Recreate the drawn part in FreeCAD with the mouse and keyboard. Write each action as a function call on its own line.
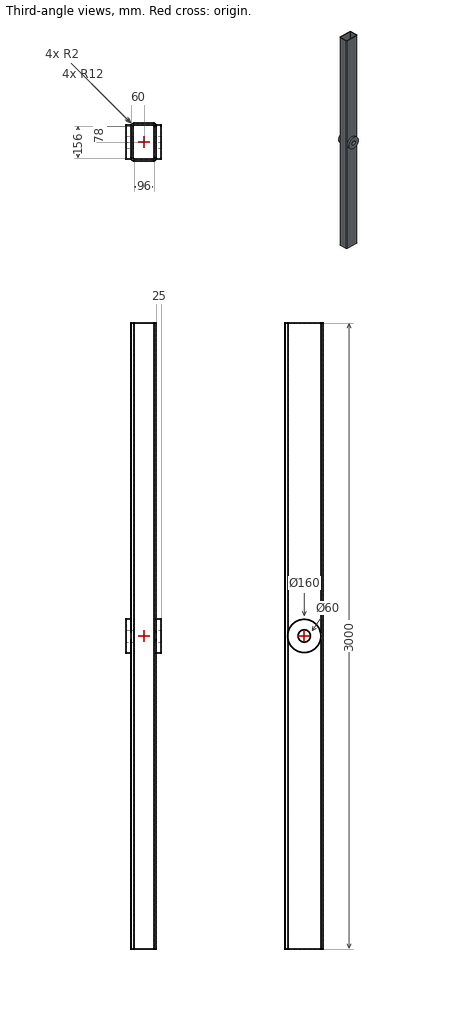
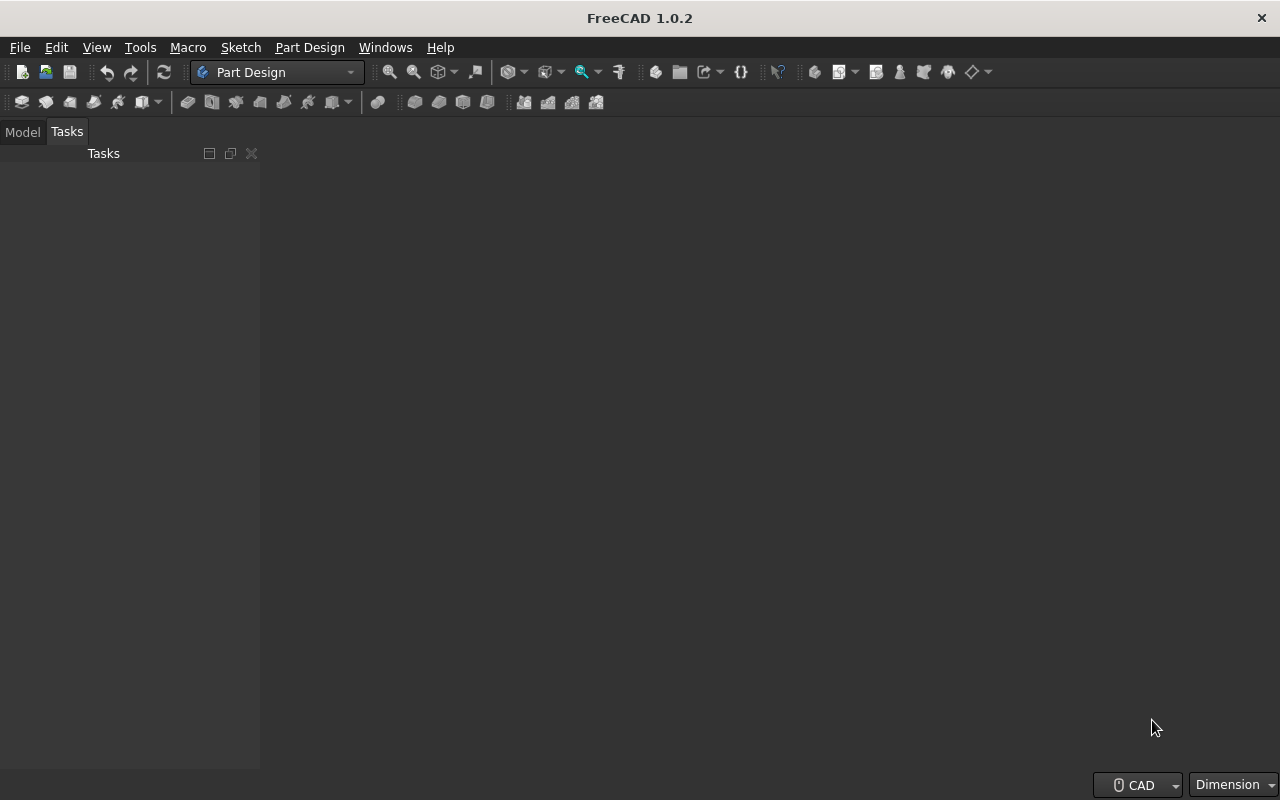
click(22, 72)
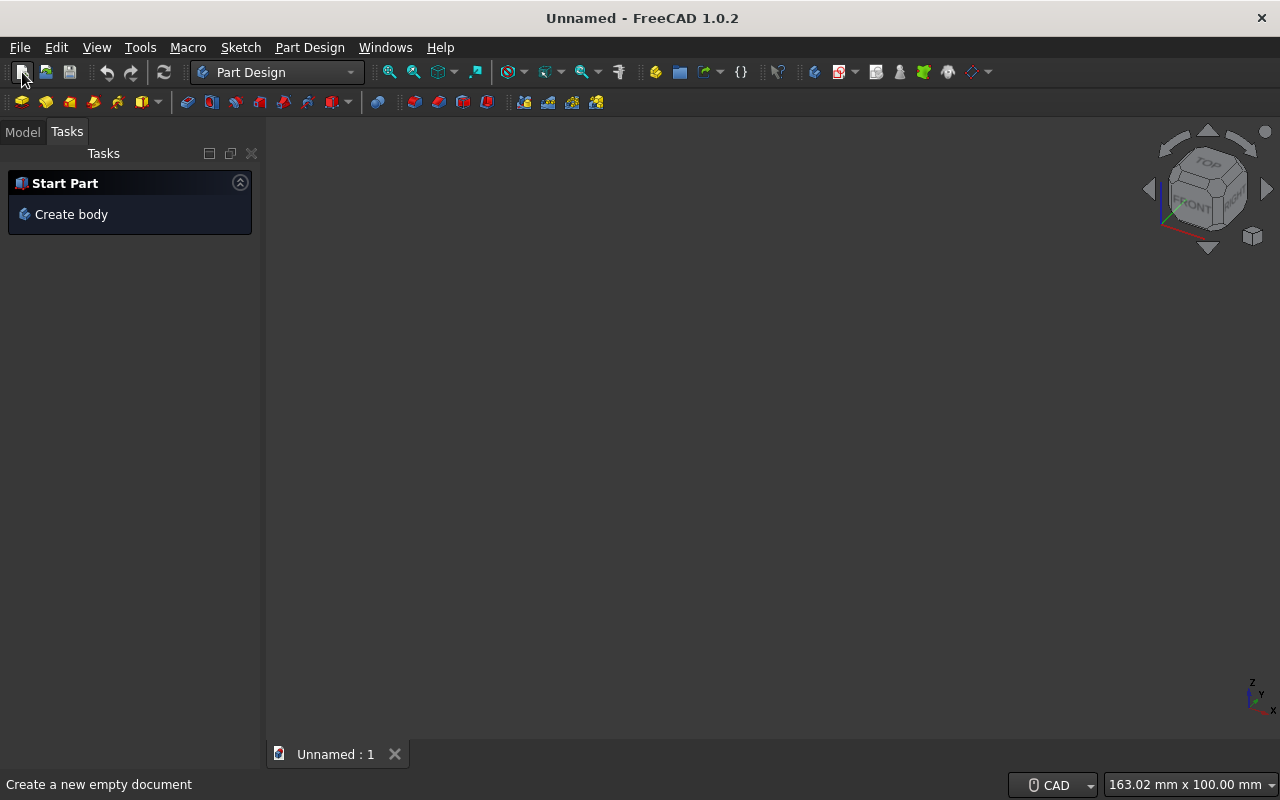
click(840, 72)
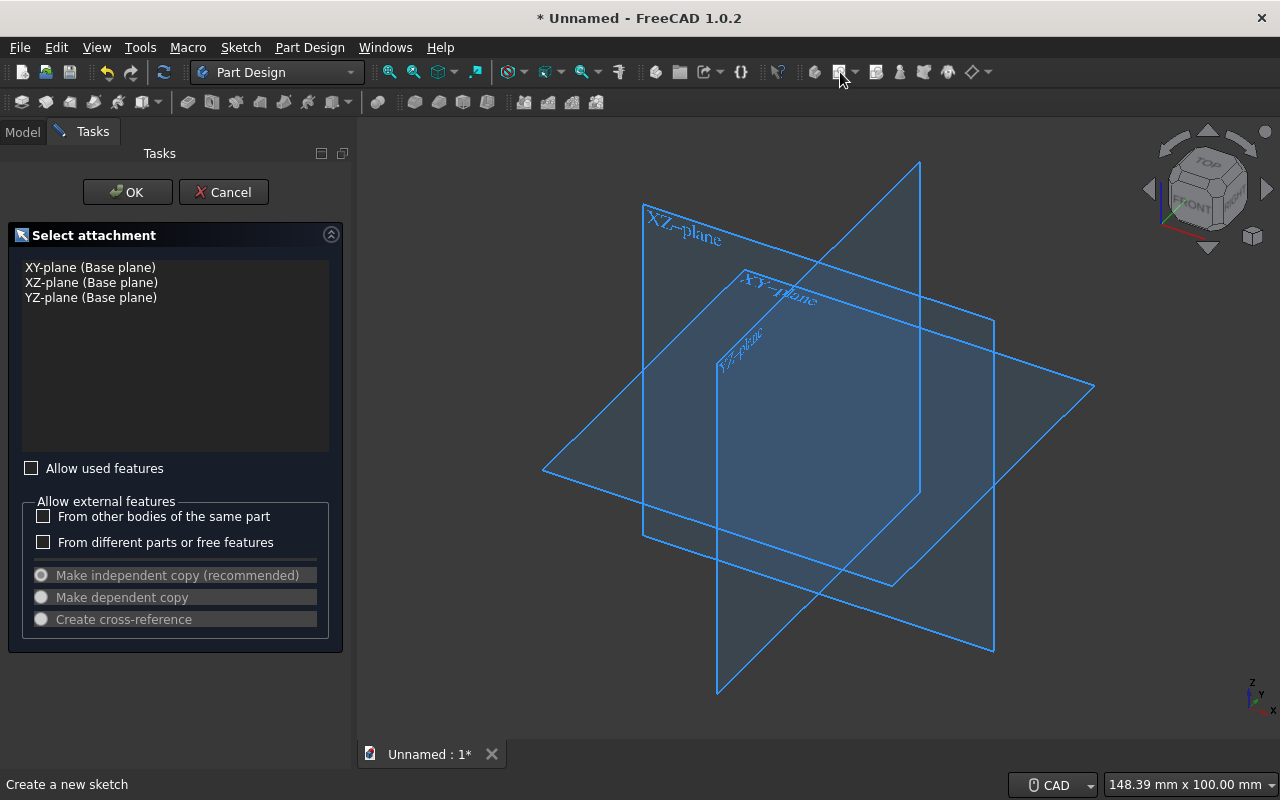
click(82, 268)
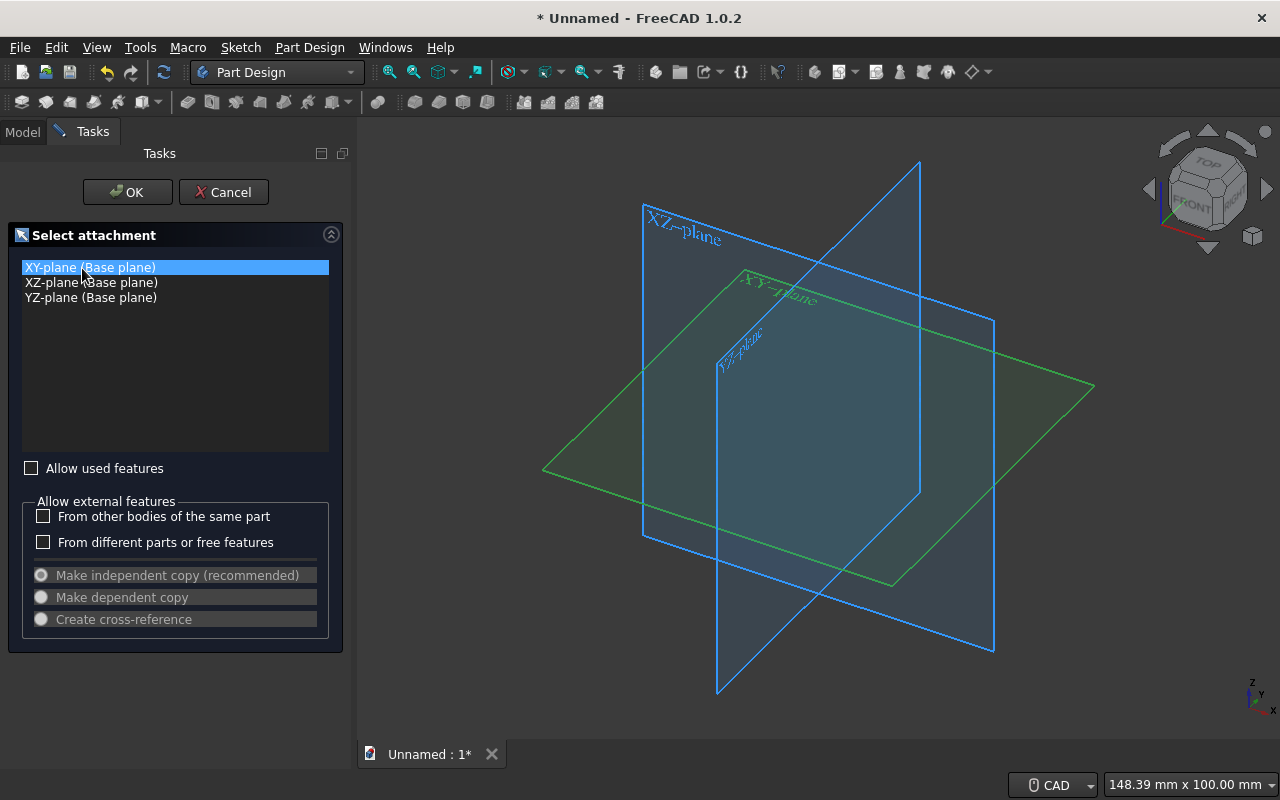
click(128, 192)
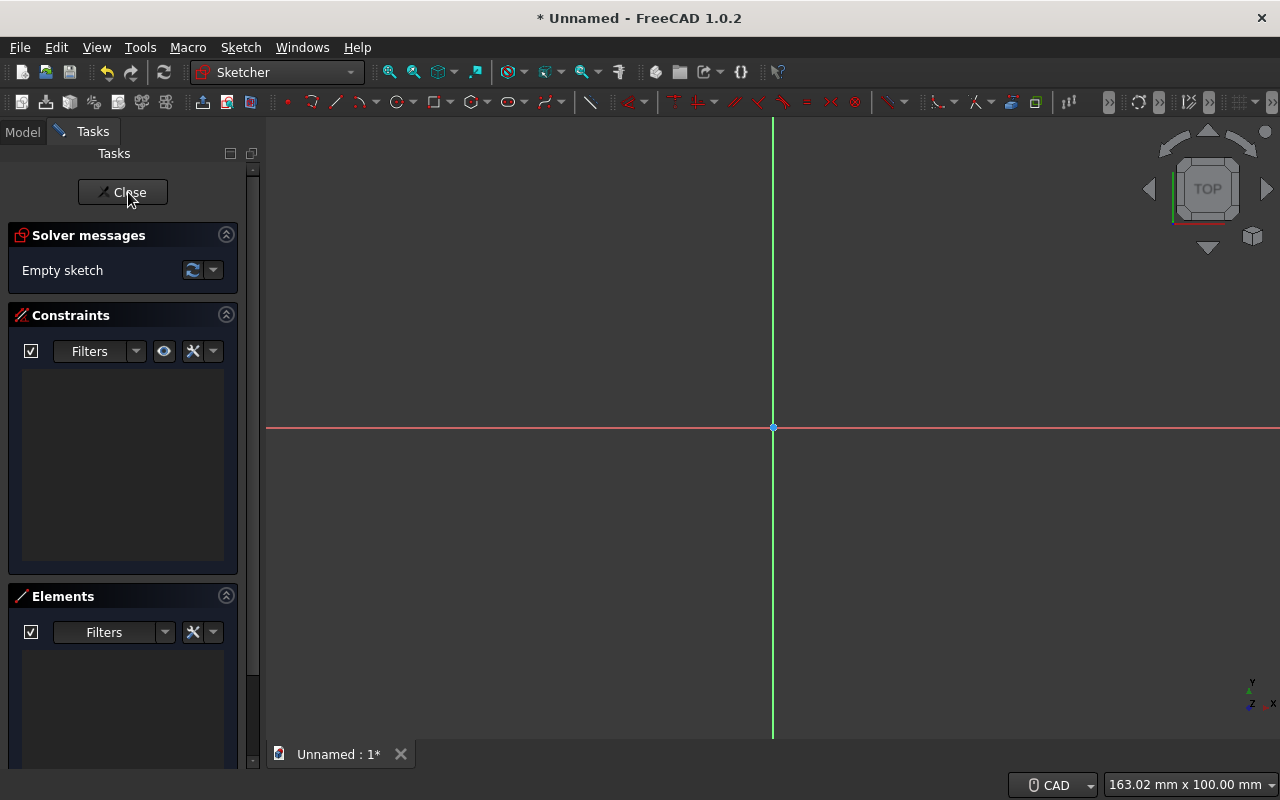
scroll(665, 428, down, 5)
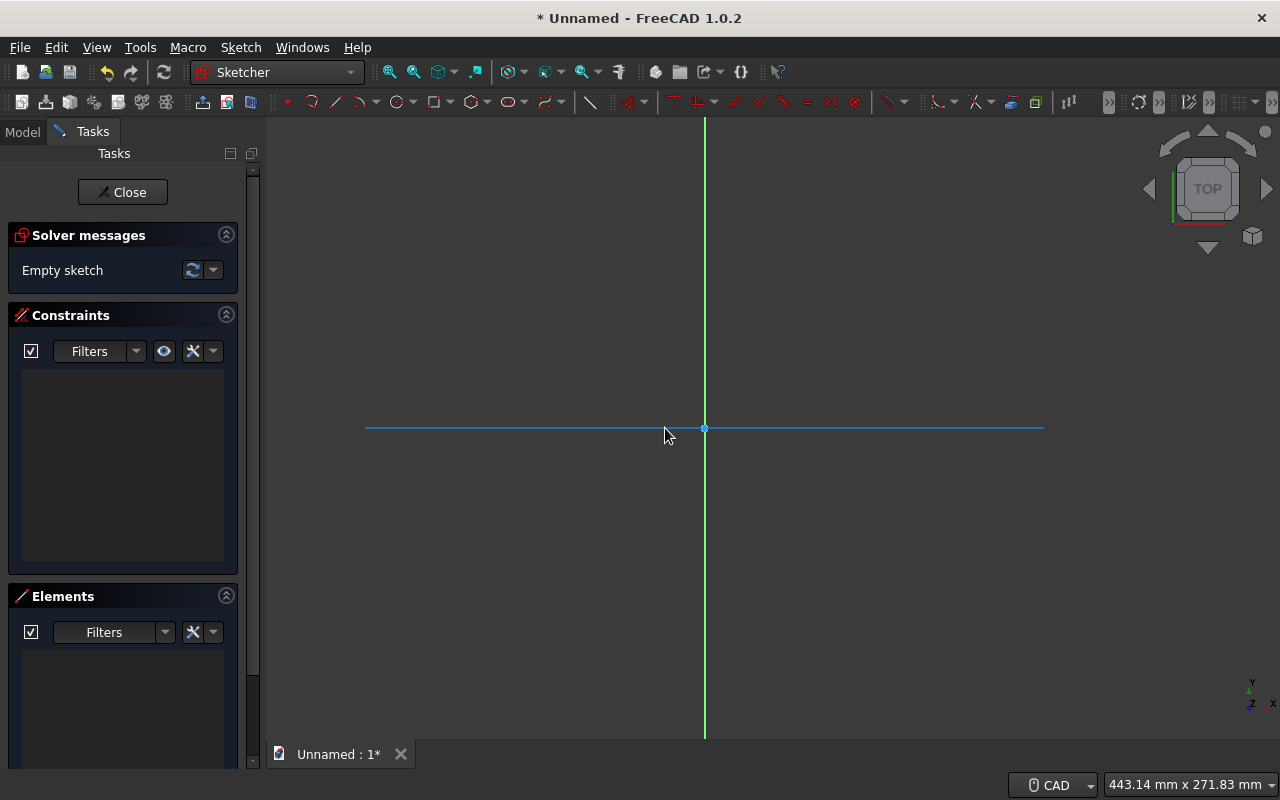
click(336, 102)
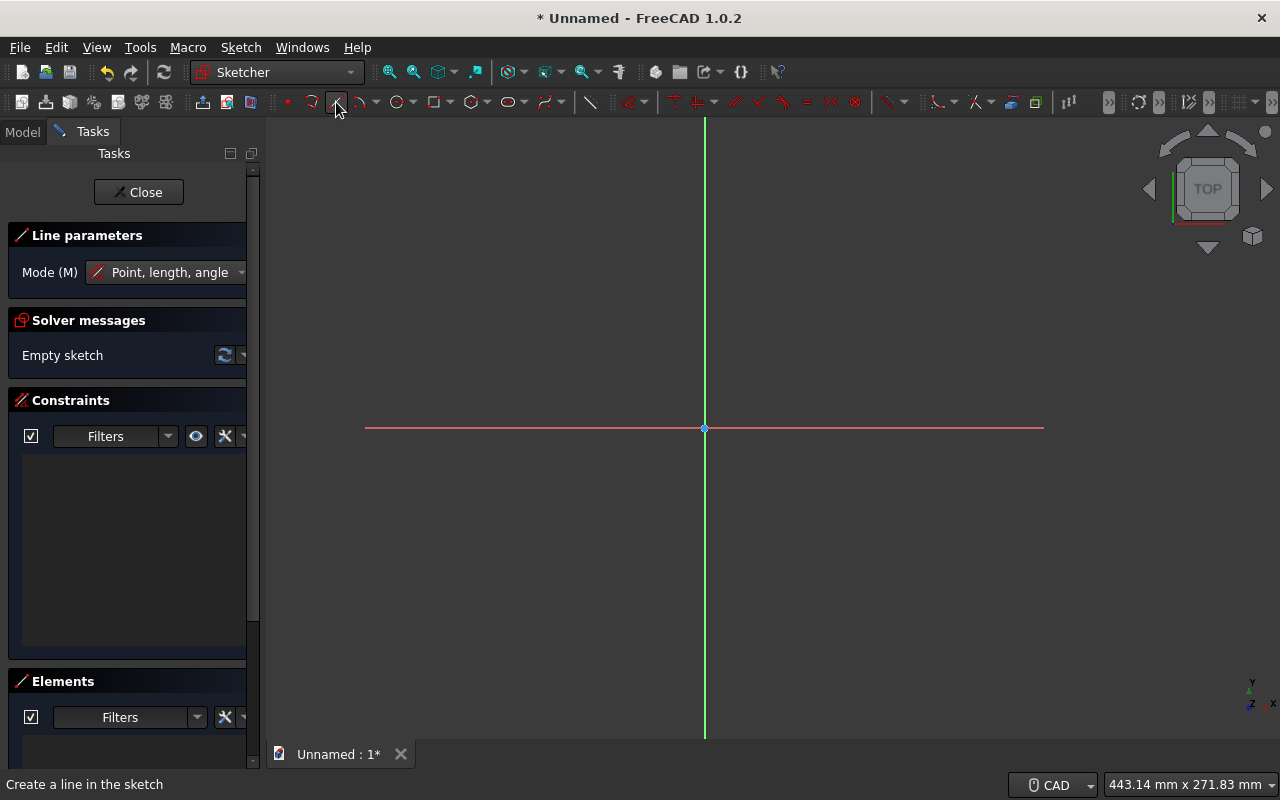
click(568, 250)
click(568, 607)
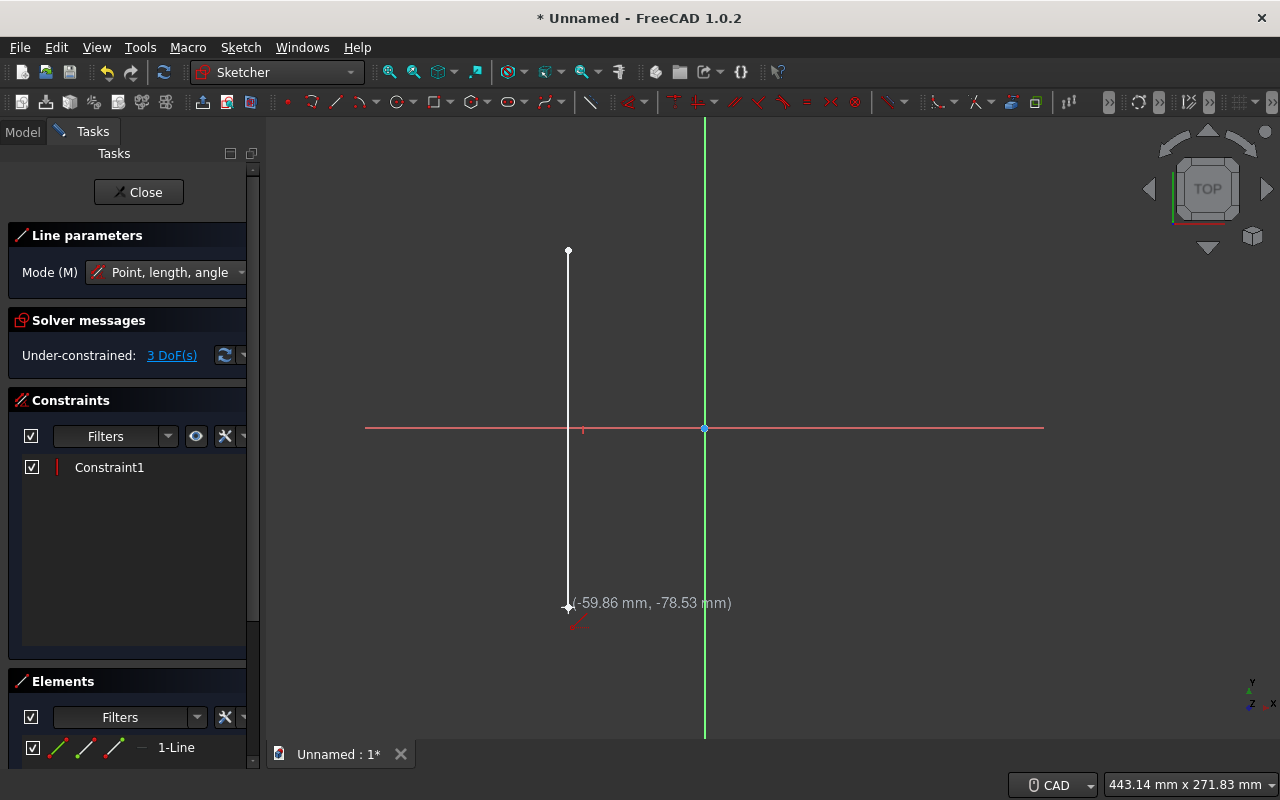
click(595, 634)
click(815, 634)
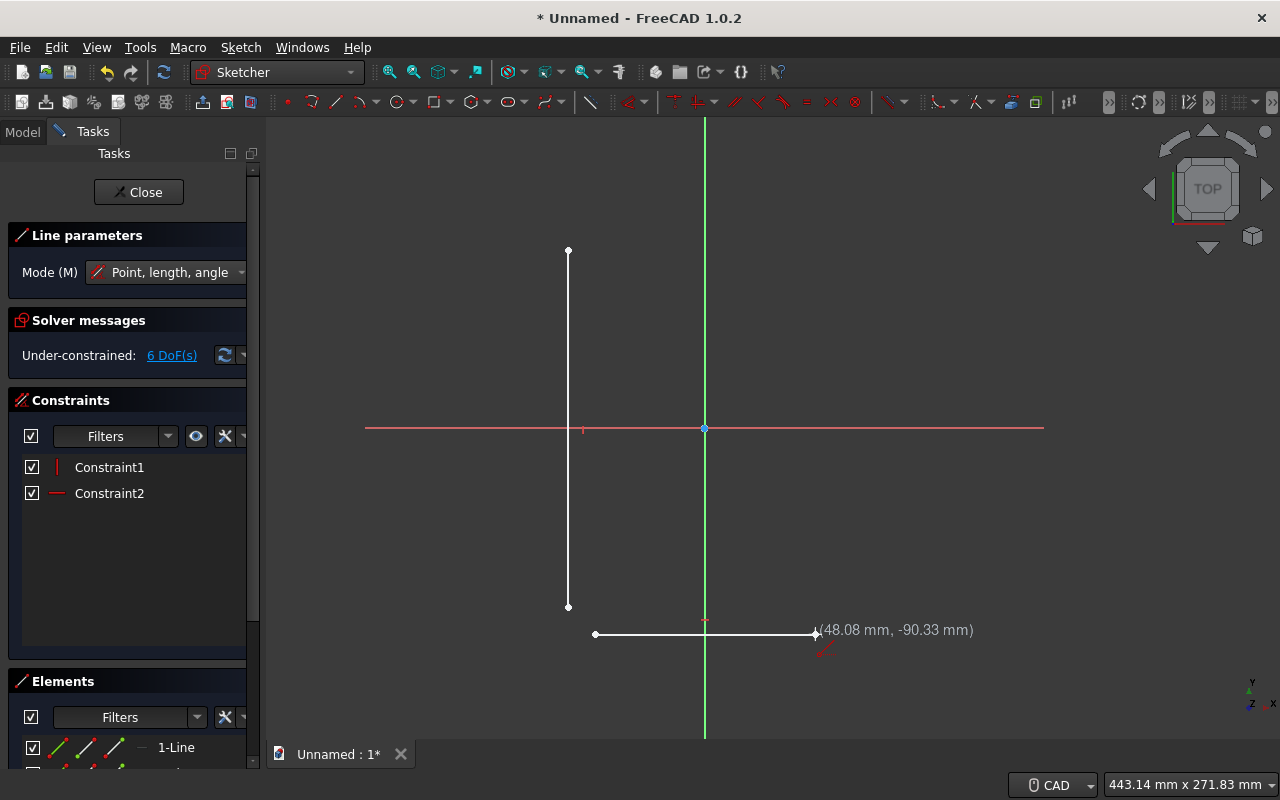
click(842, 607)
click(842, 250)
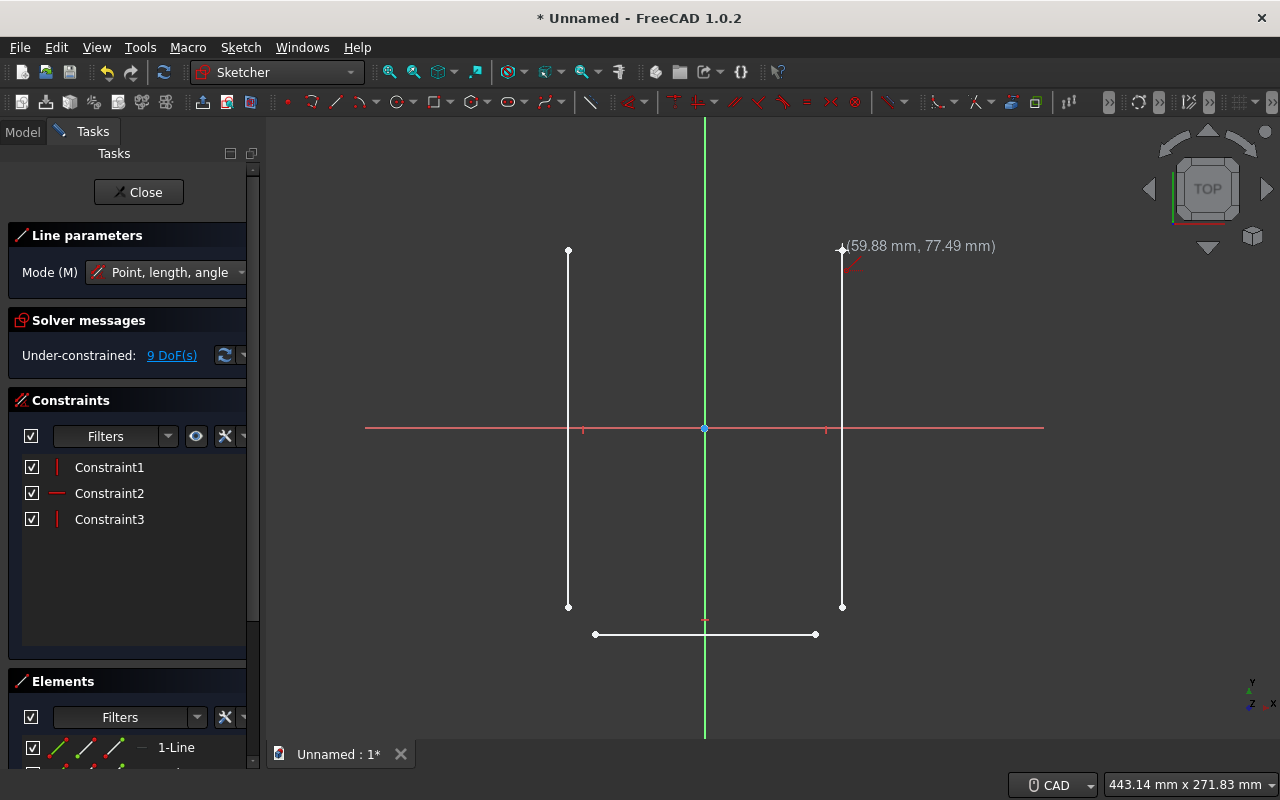
click(815, 222)
click(595, 222)